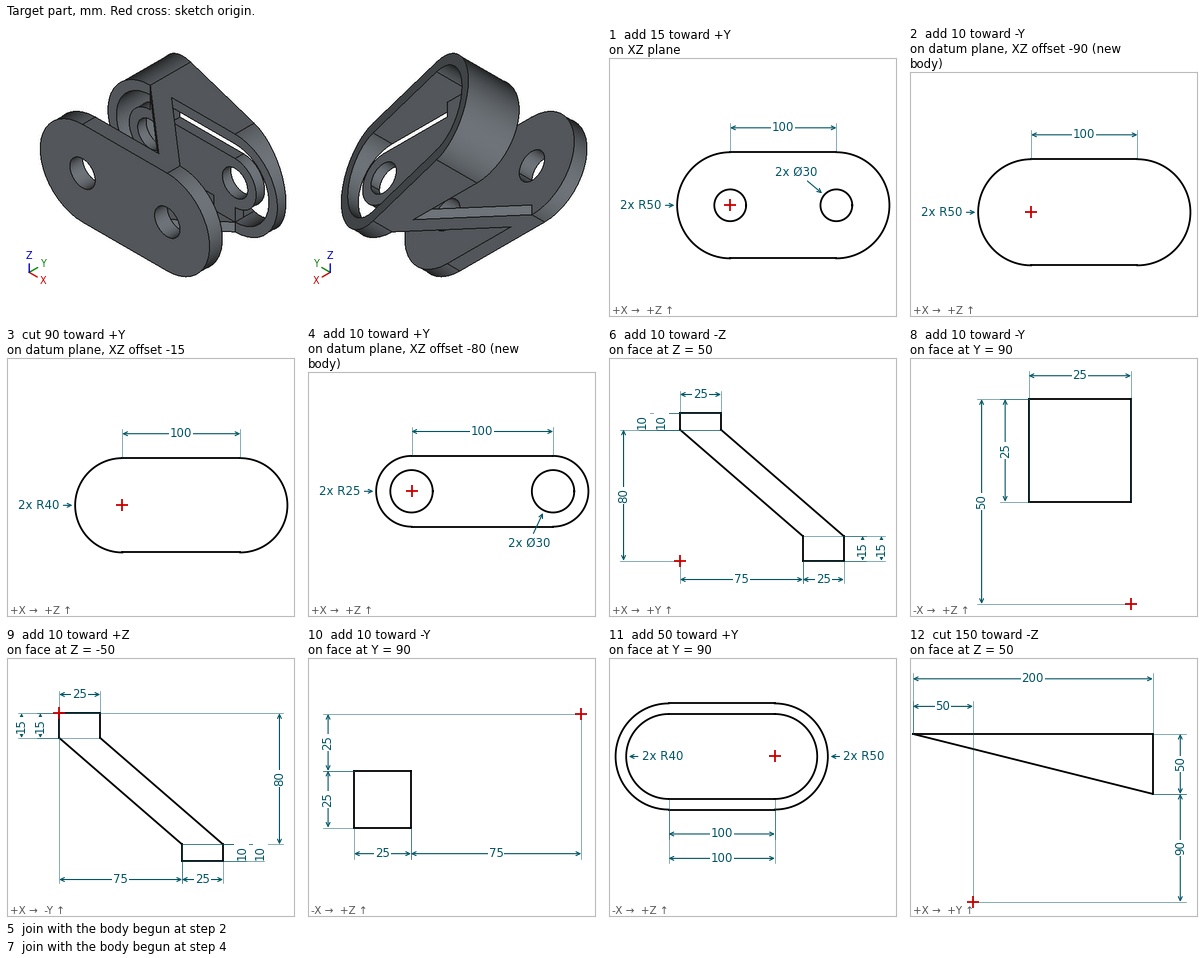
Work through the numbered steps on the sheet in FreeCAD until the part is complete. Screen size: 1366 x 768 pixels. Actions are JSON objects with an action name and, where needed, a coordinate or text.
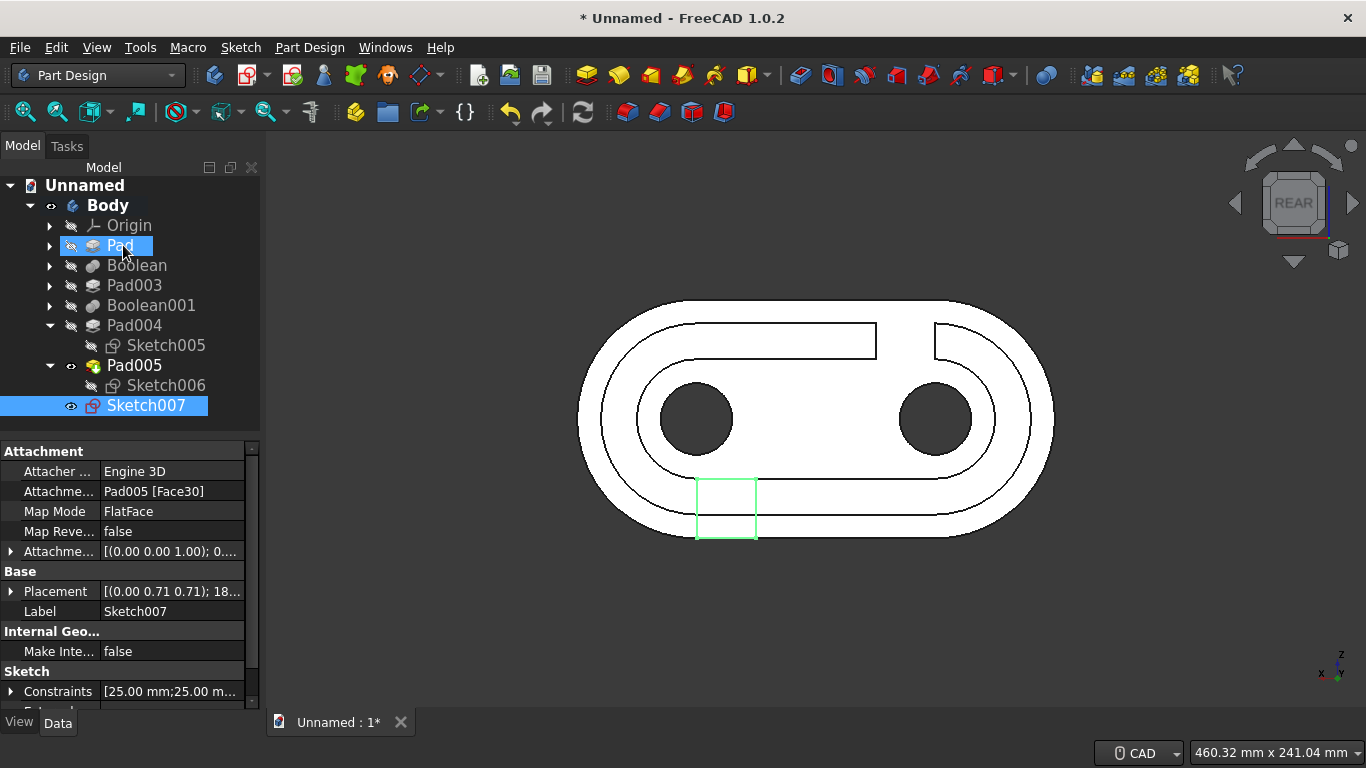
{"action": "left_click", "coordinate": [588, 76]}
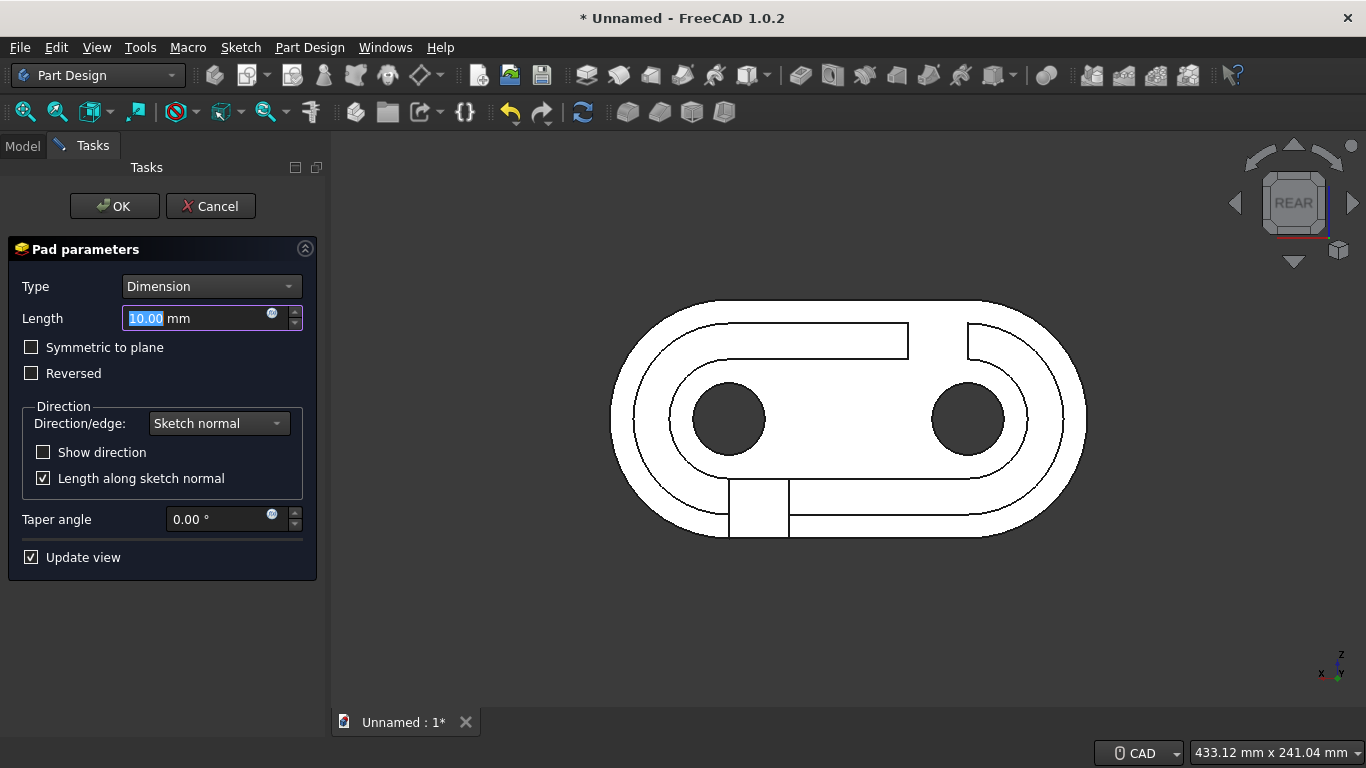
{"action": "type", "text": "10"}
{"action": "key", "text": "Tab"}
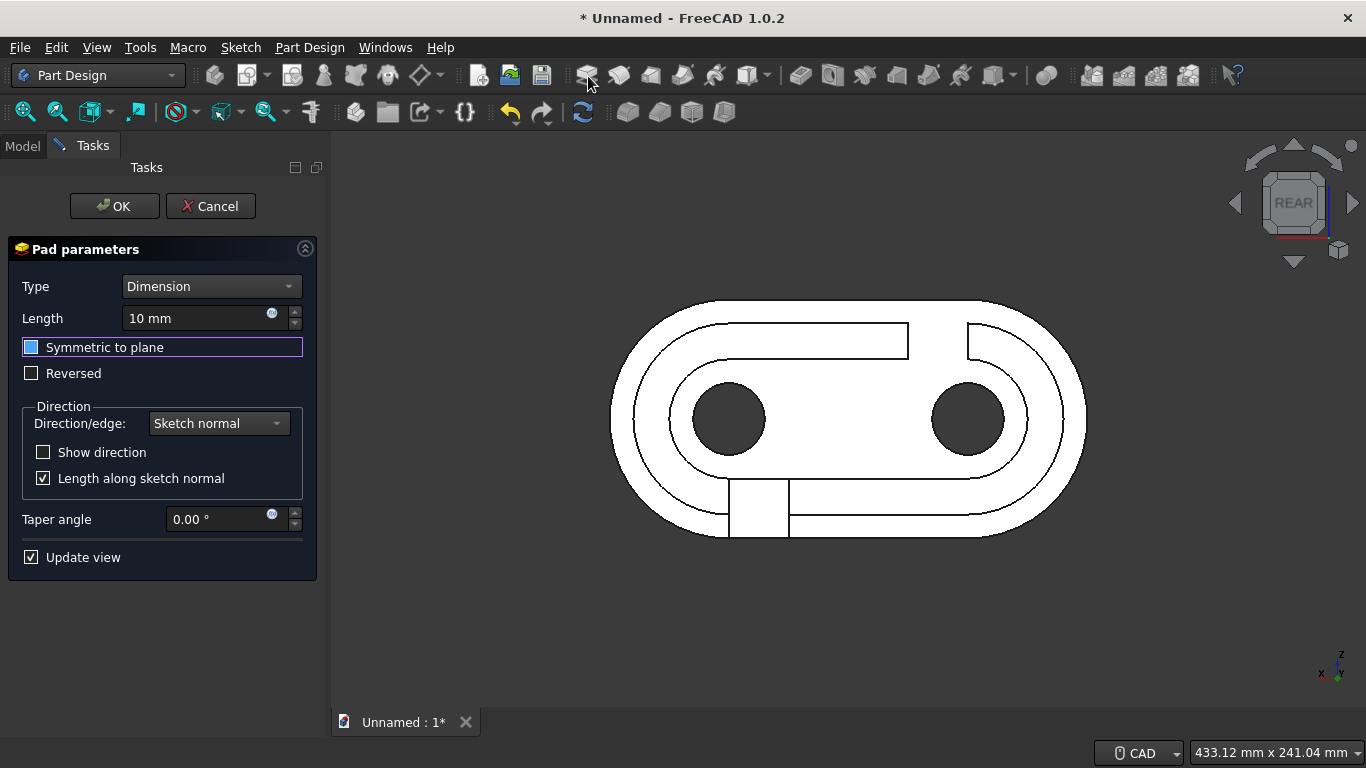
{"action": "left_click", "coordinate": [30, 373]}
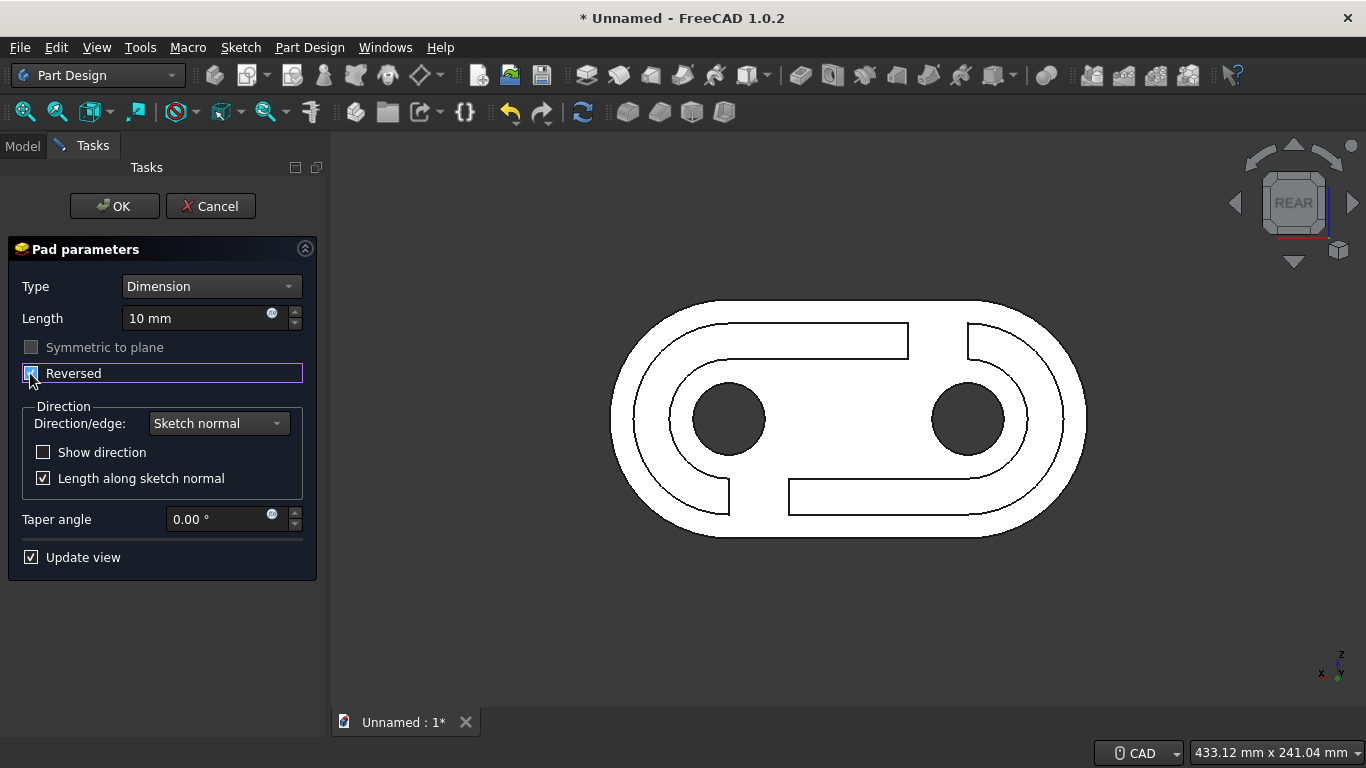
{"action": "left_click", "coordinate": [115, 206]}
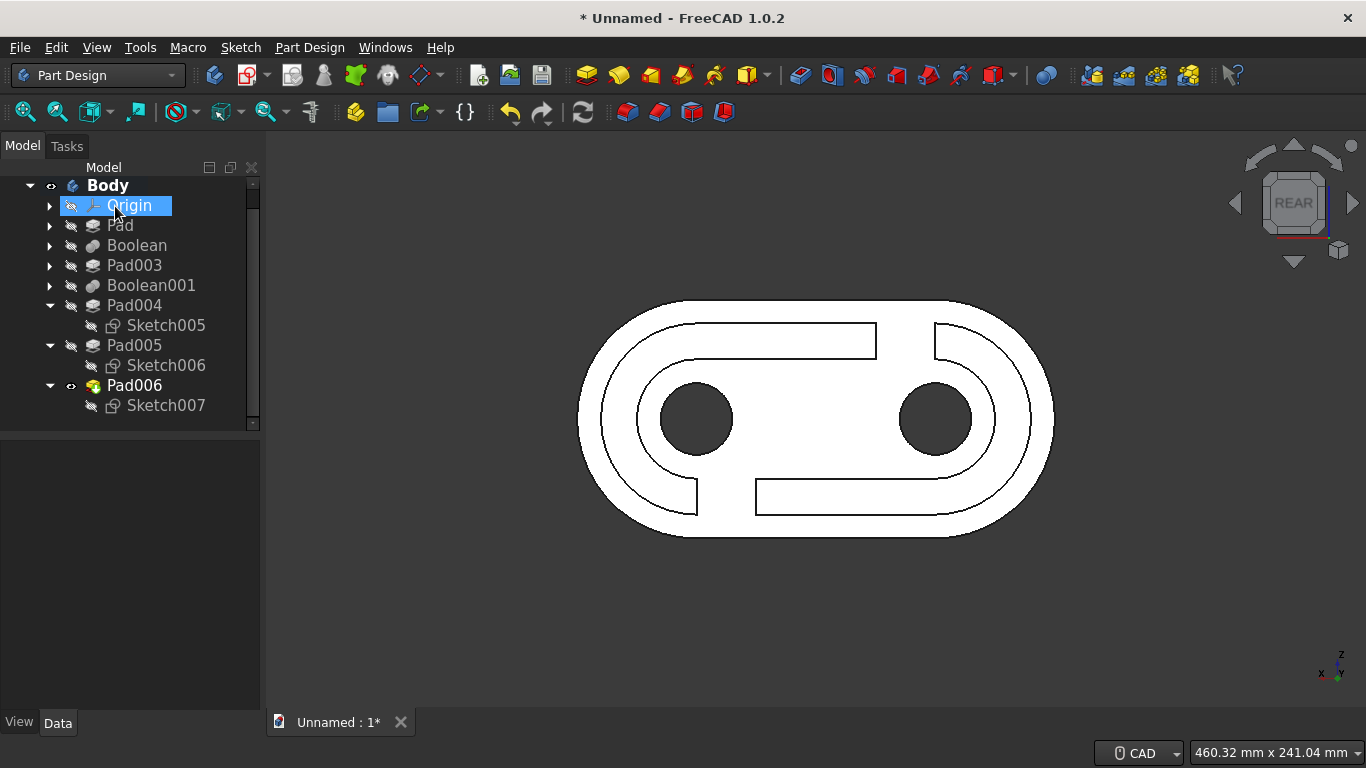
{"action": "left_click", "coordinate": [26, 112]}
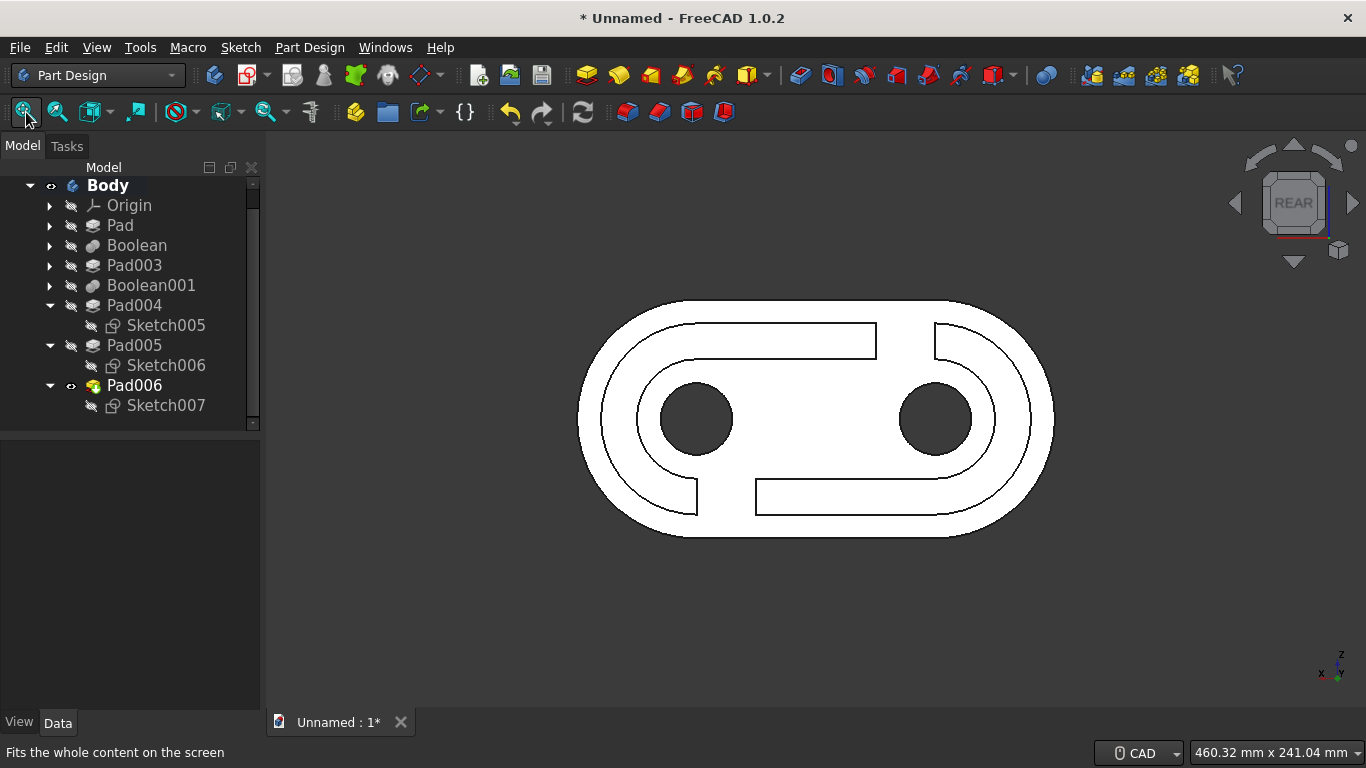
{"action": "left_click", "coordinate": [816, 418]}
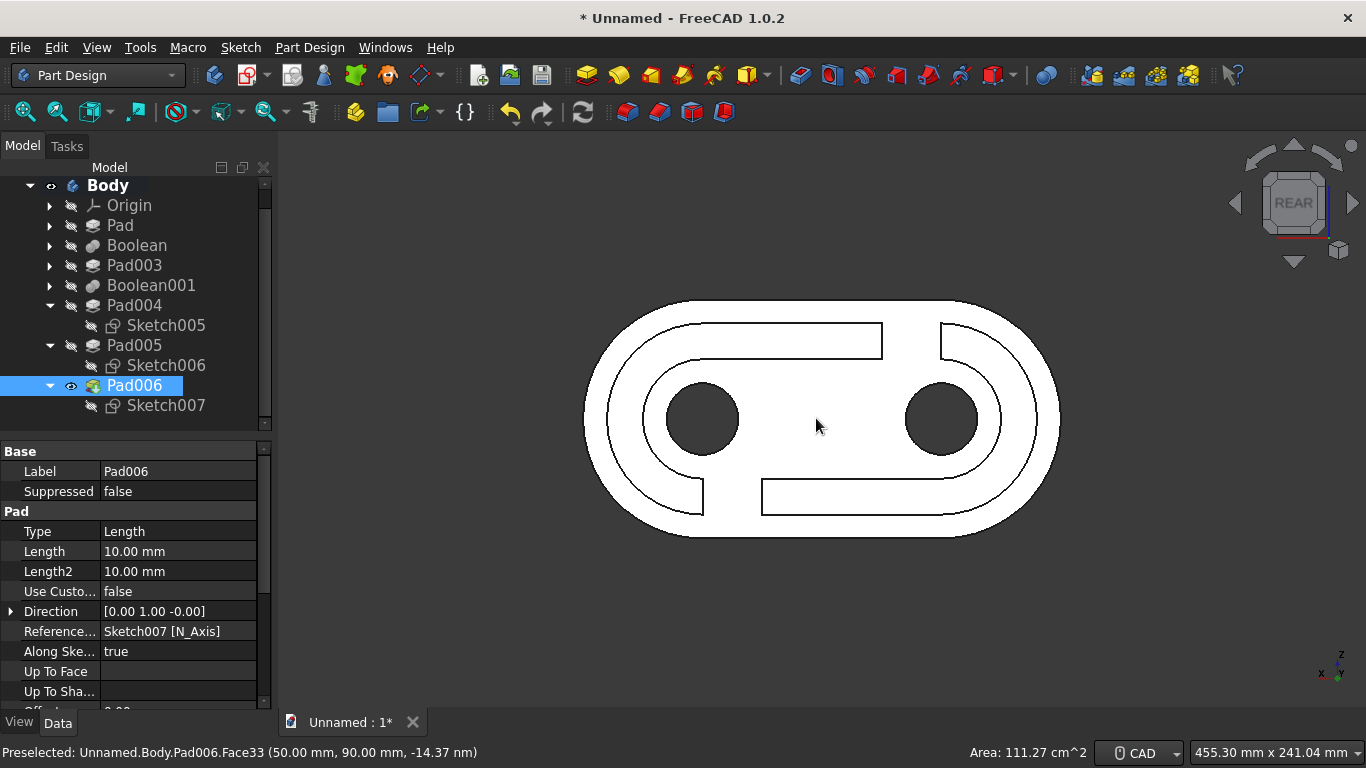
{"action": "left_click", "coordinate": [248, 76]}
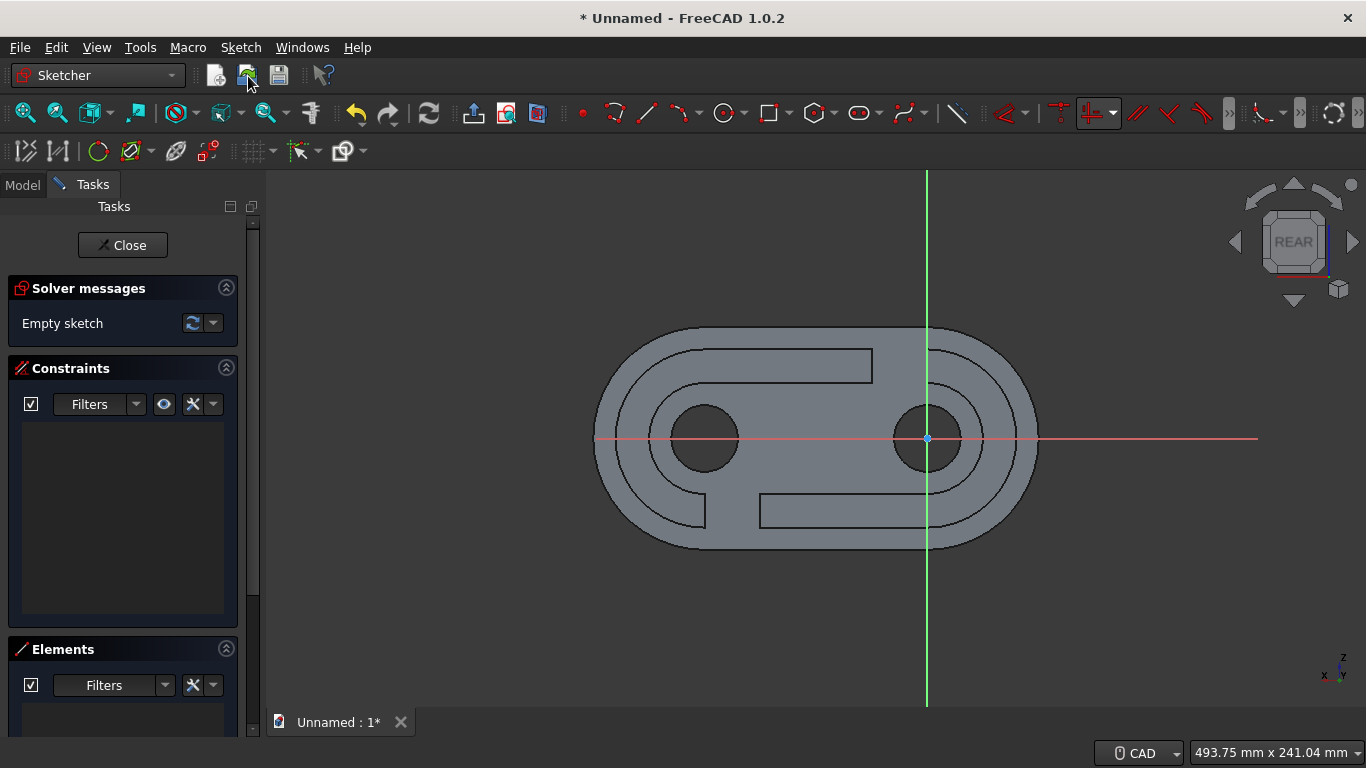
{"action": "scroll", "coordinate": [955, 439], "scroll_direction": "up", "scroll_amount": 2}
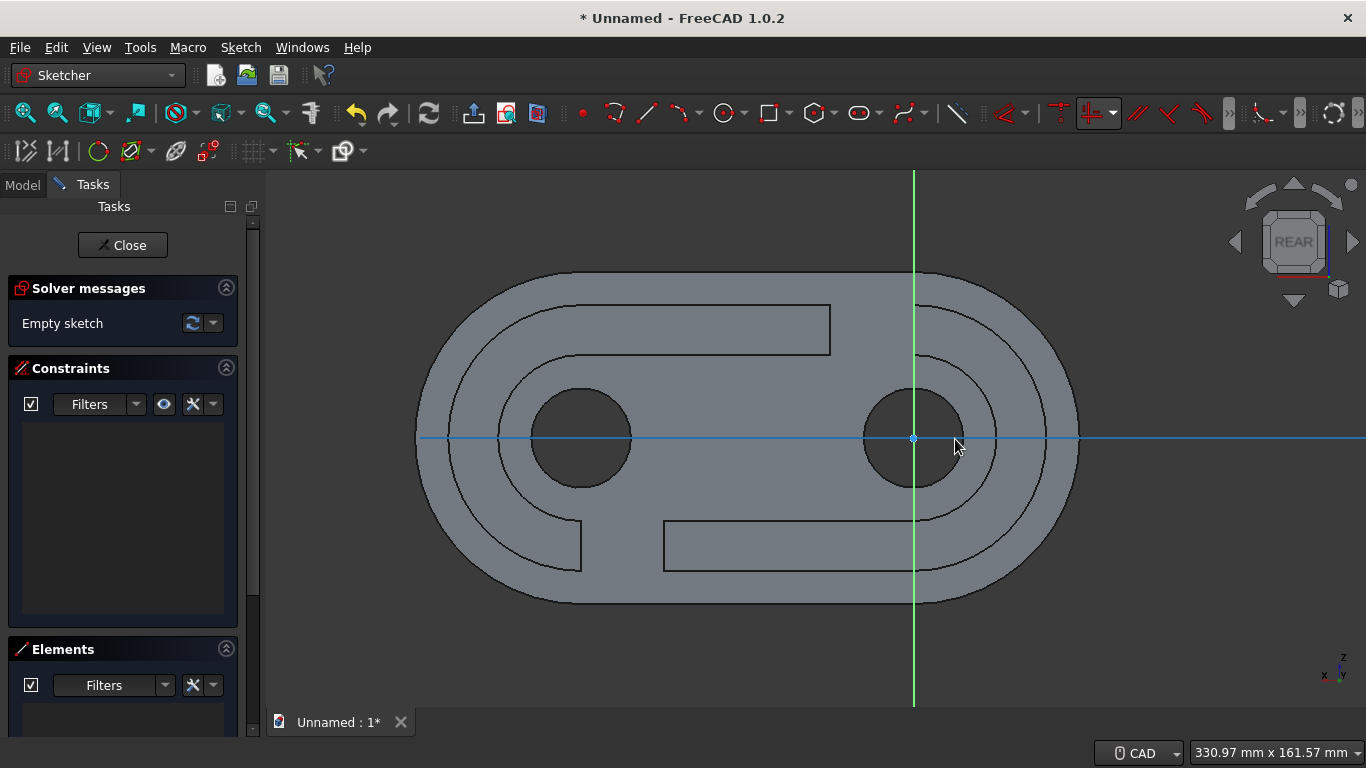
{"action": "left_click", "coordinate": [860, 114]}